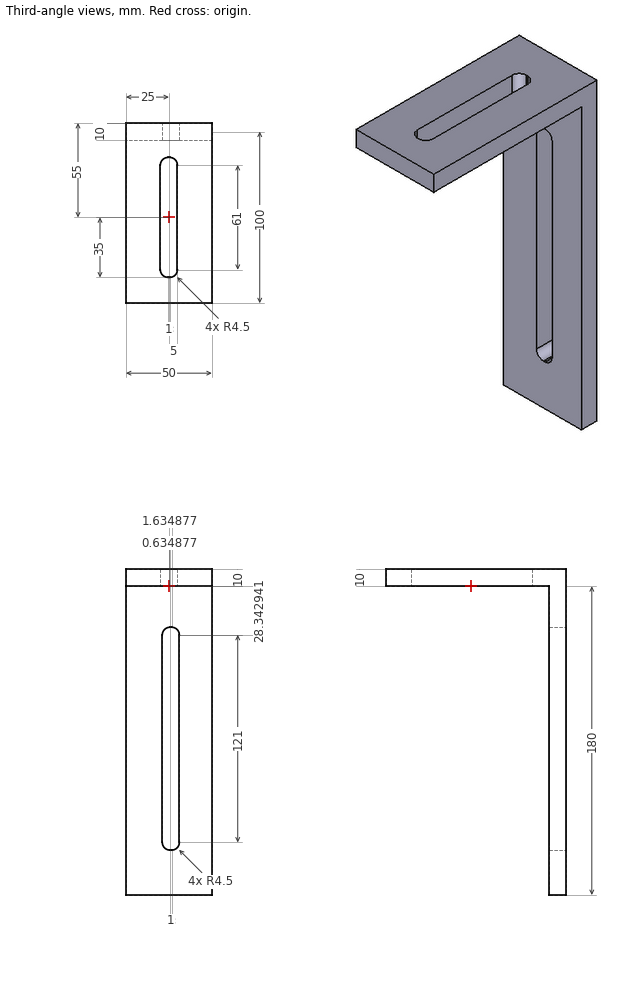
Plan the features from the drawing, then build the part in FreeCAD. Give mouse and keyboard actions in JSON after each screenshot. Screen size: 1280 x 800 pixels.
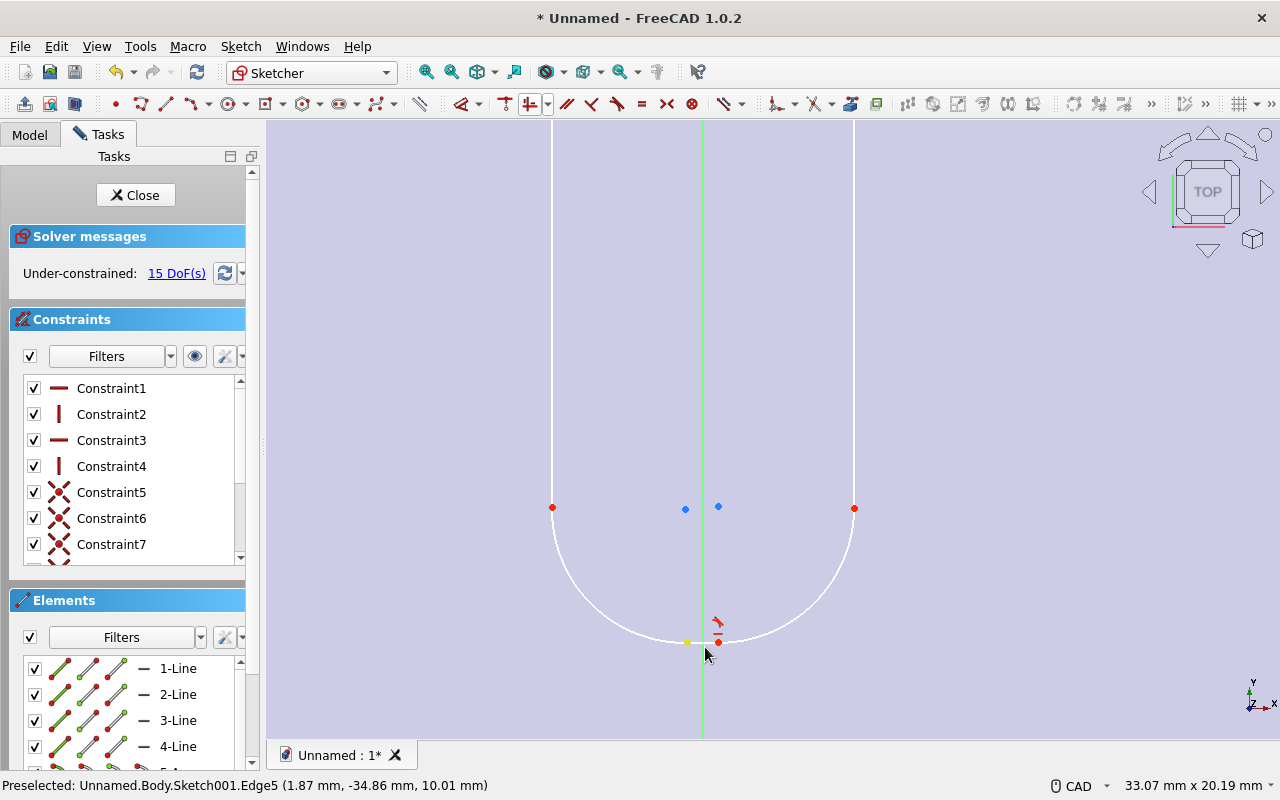
{"action": "left_click", "coordinate": [703, 643]}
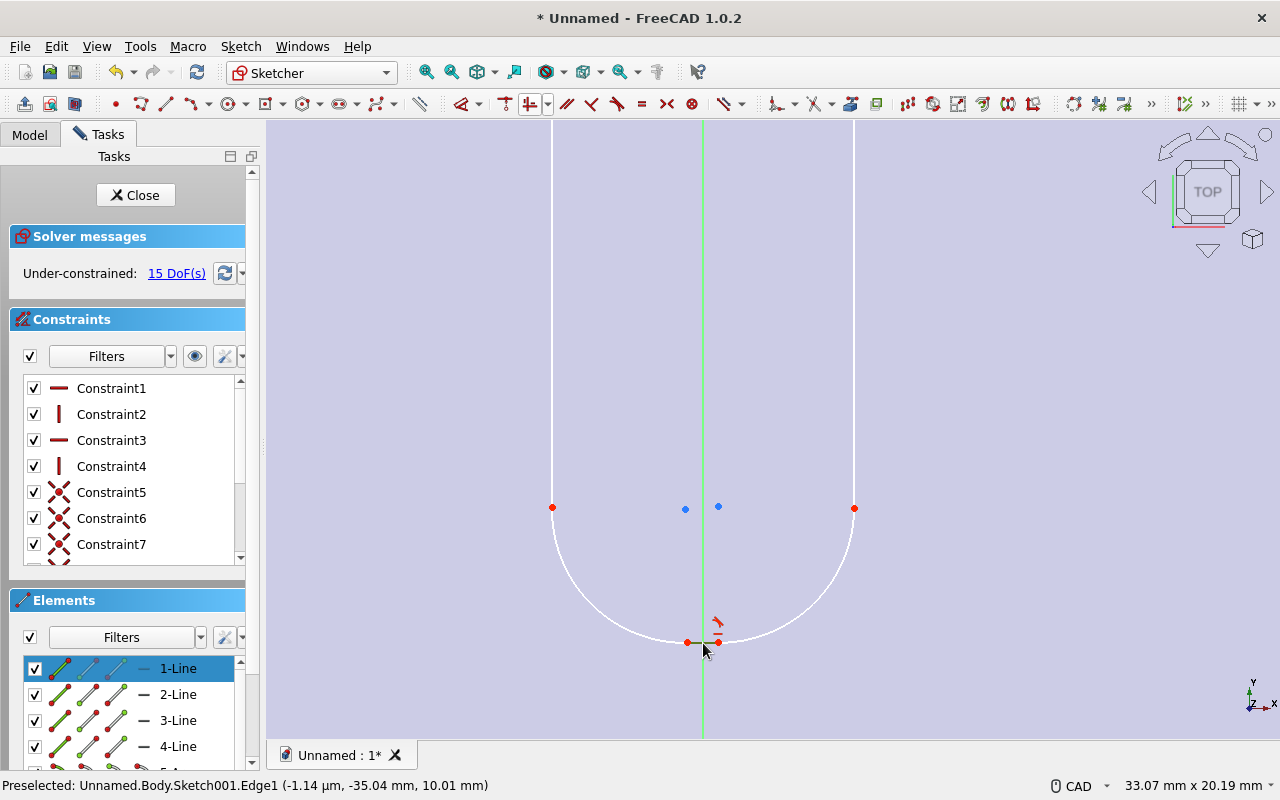
{"action": "scroll", "coordinate": [705, 647], "scroll_direction": "down", "scroll_amount": 8}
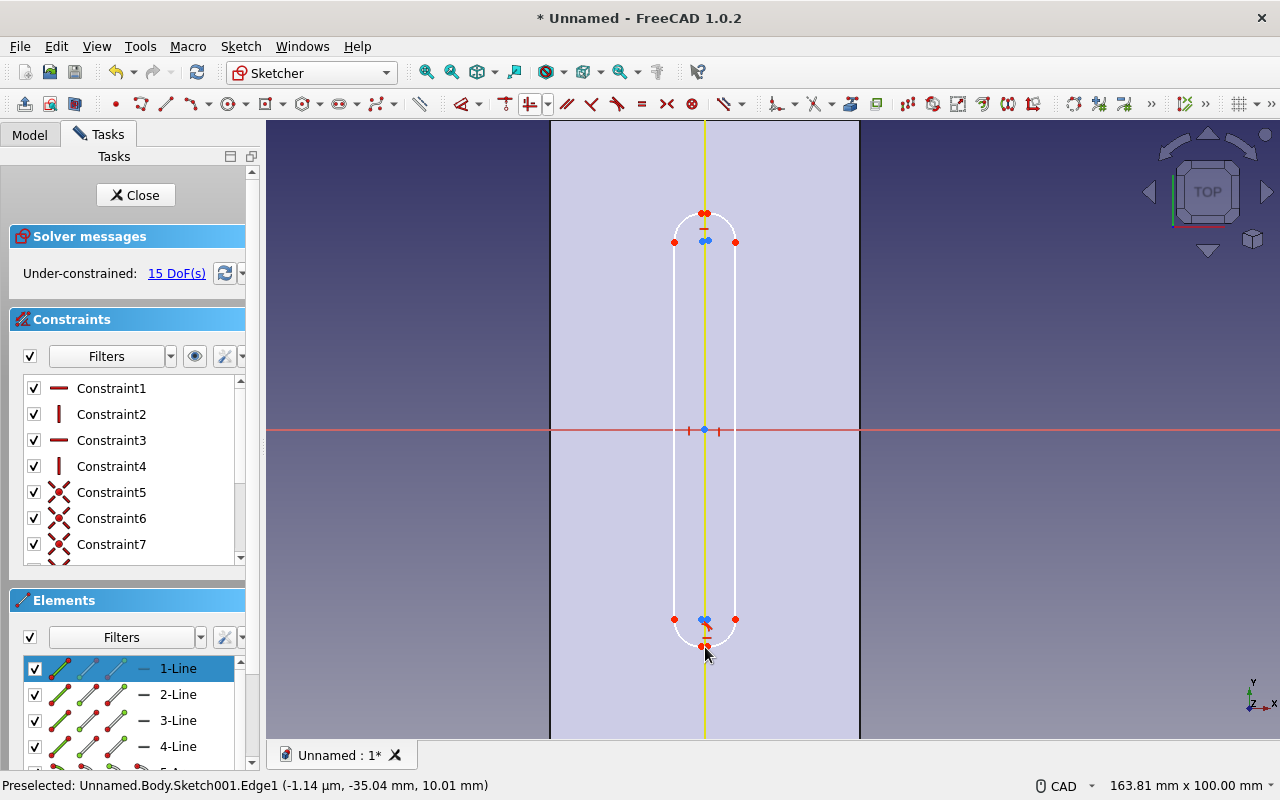
{"action": "left_click", "coordinate": [677, 632]}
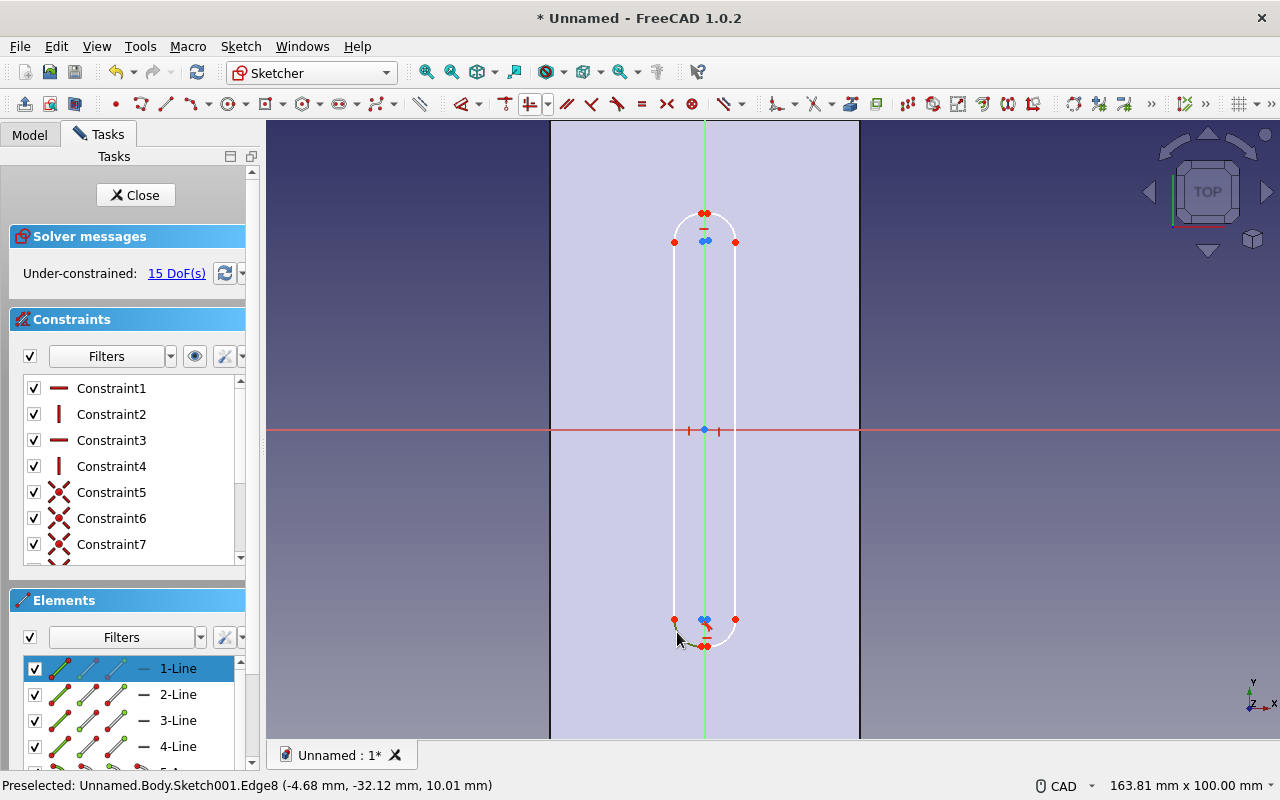
{"action": "left_click", "coordinate": [617, 104]}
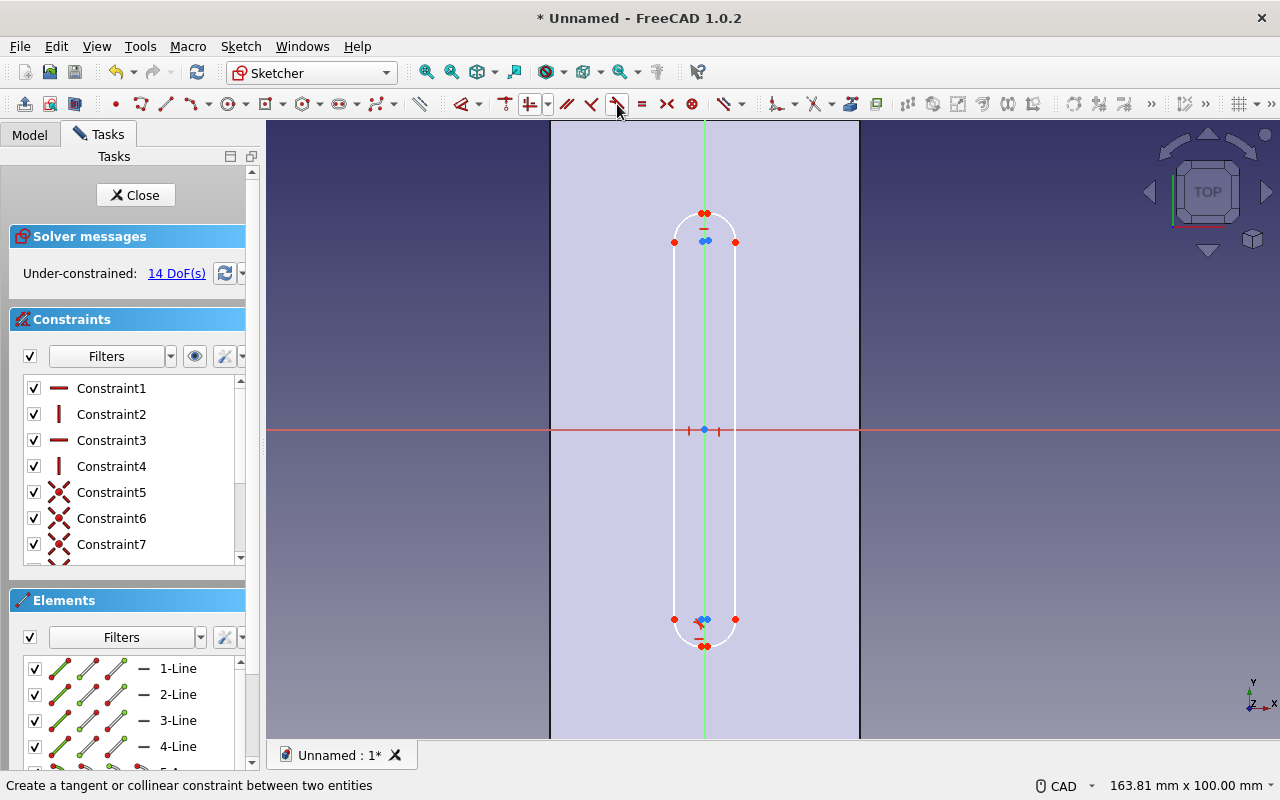
{"action": "left_click", "coordinate": [735, 507]}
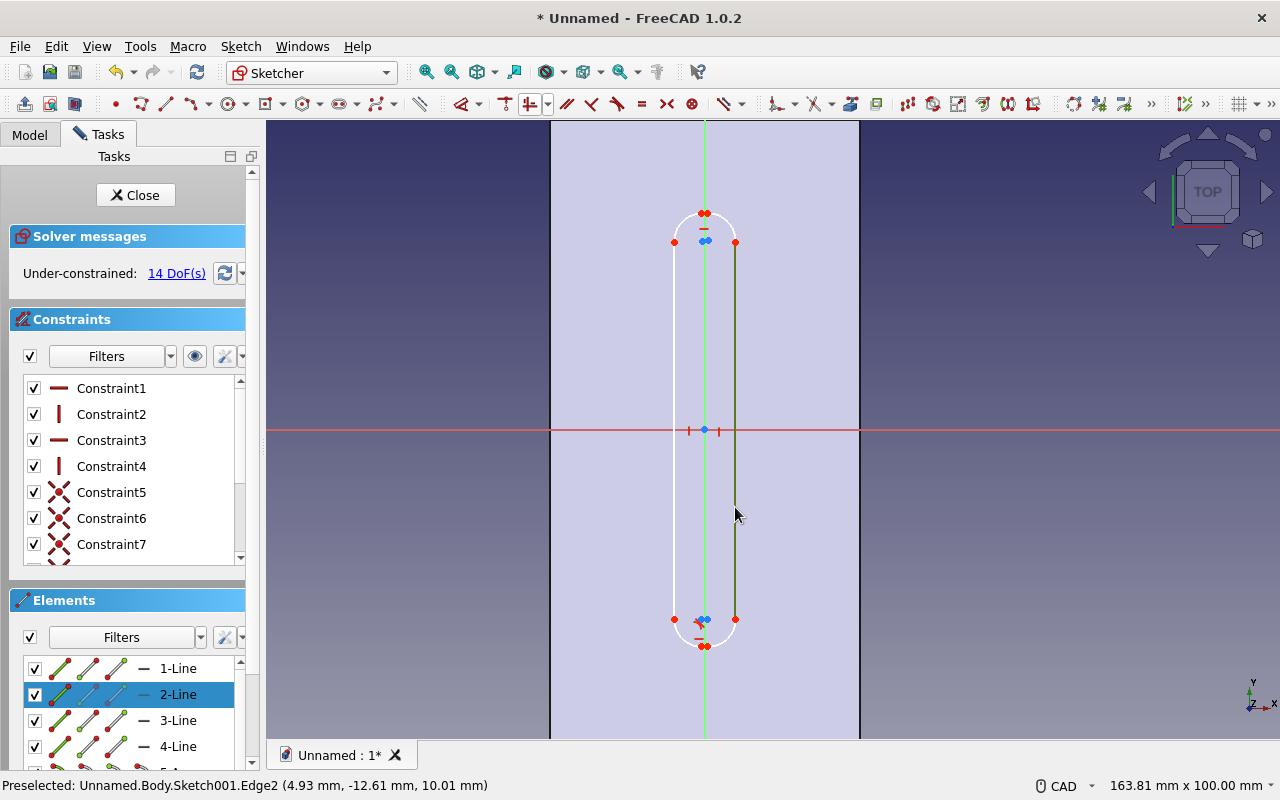
{"action": "left_click", "coordinate": [720, 644]}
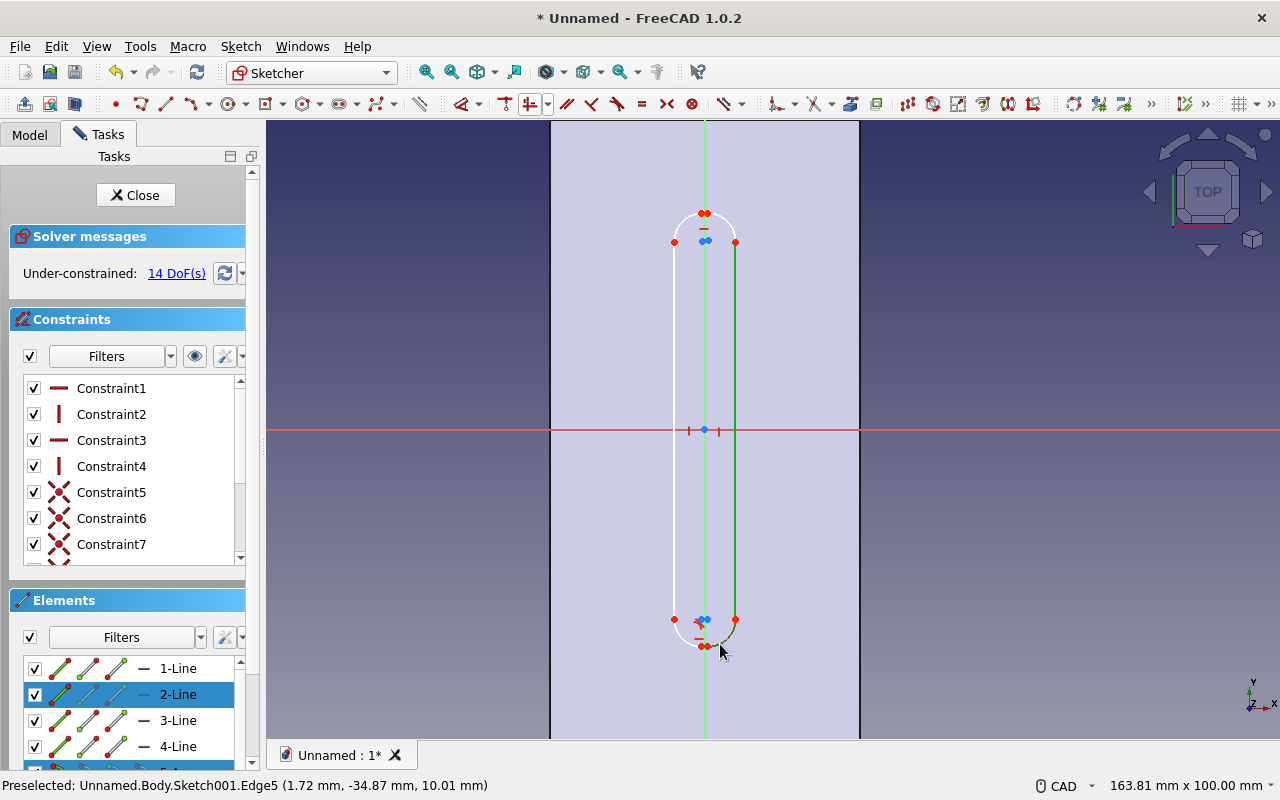
{"action": "left_click", "coordinate": [617, 104]}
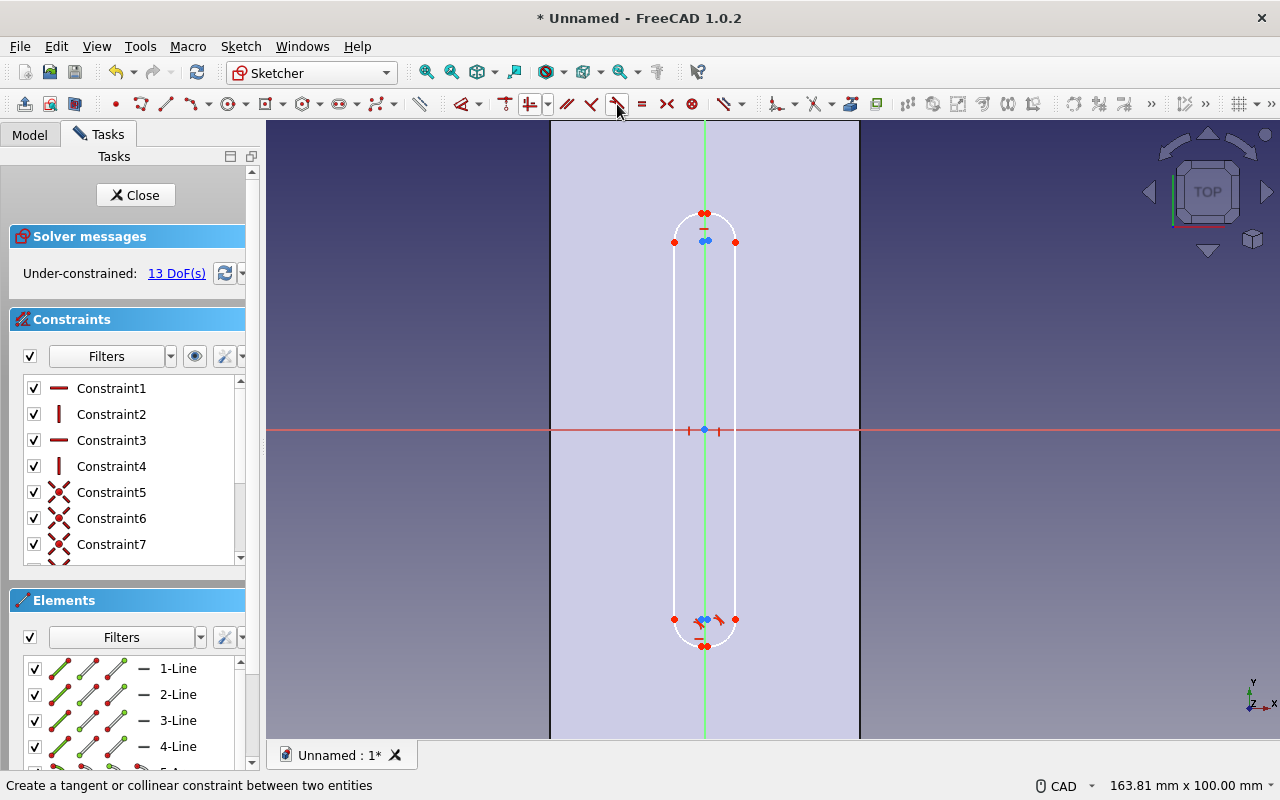
{"action": "left_click", "coordinate": [735, 506]}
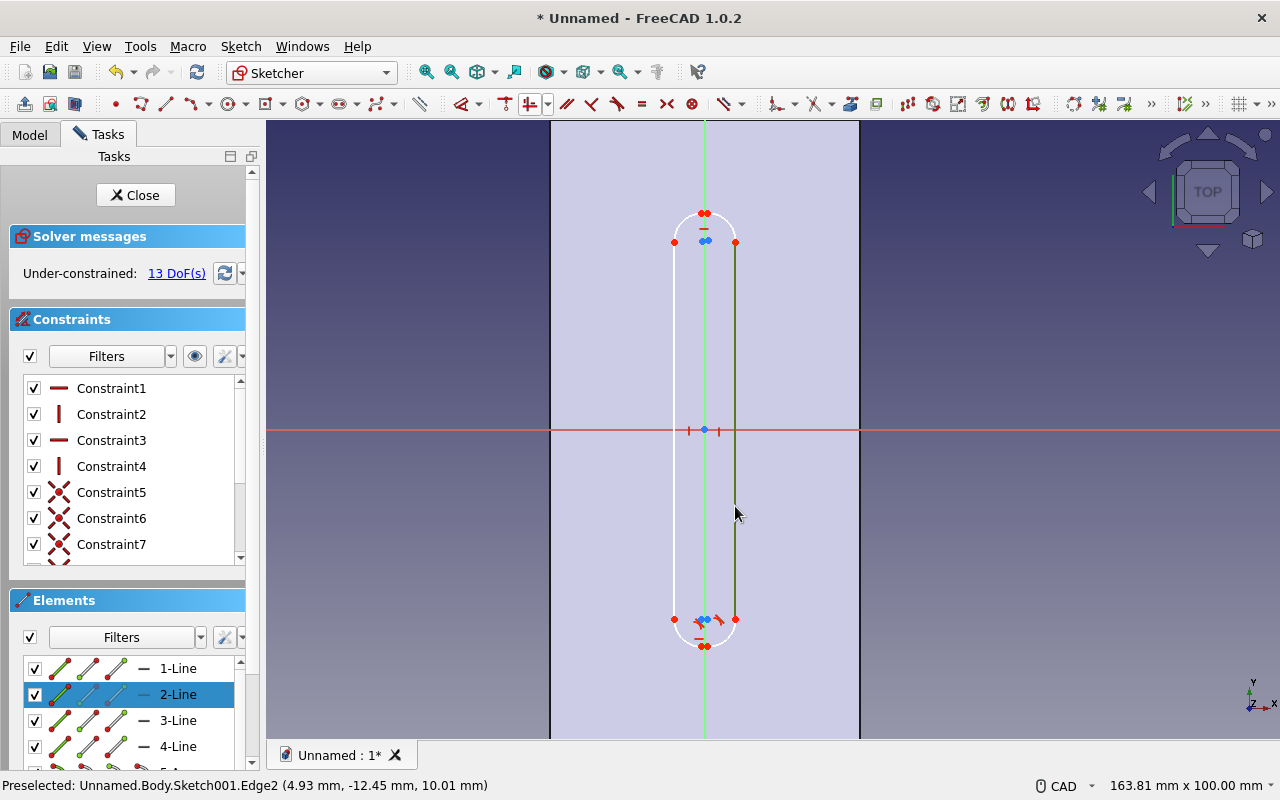
{"action": "left_click", "coordinate": [733, 229]}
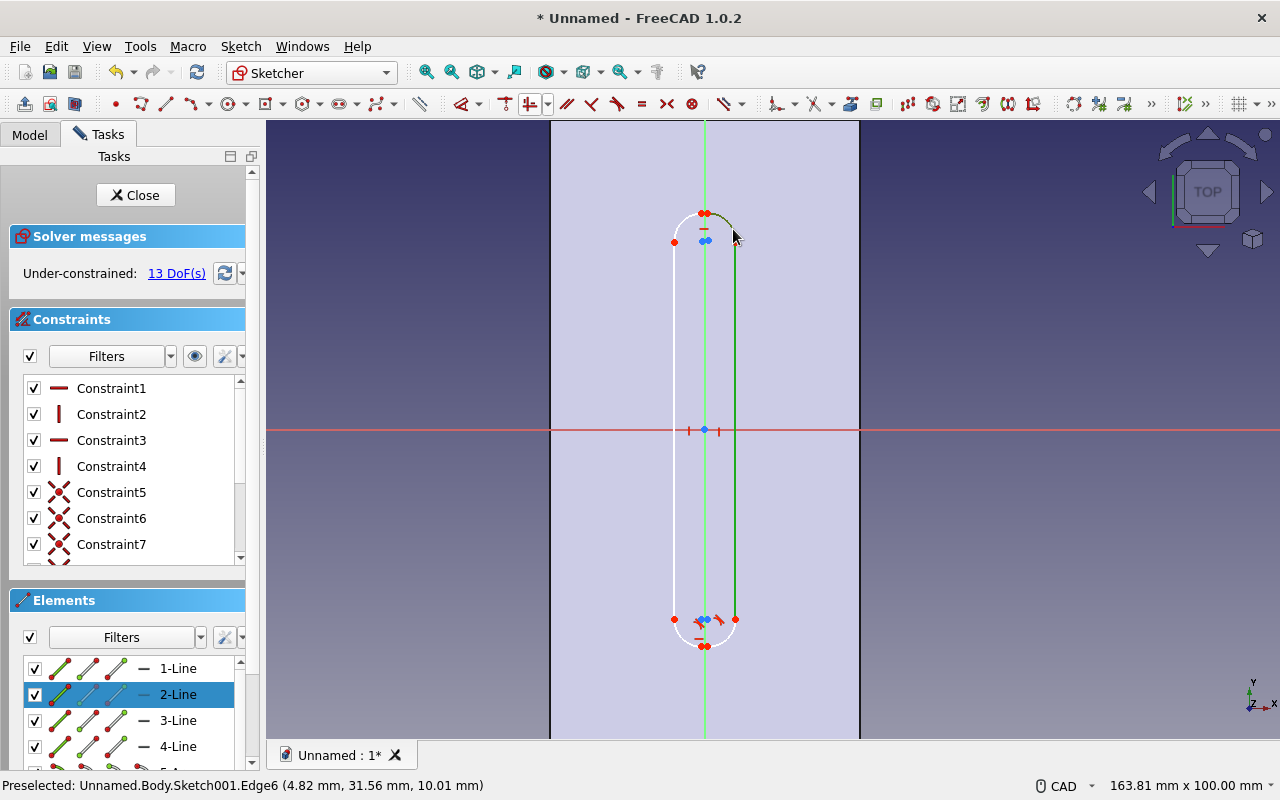
{"action": "left_click", "coordinate": [617, 104]}